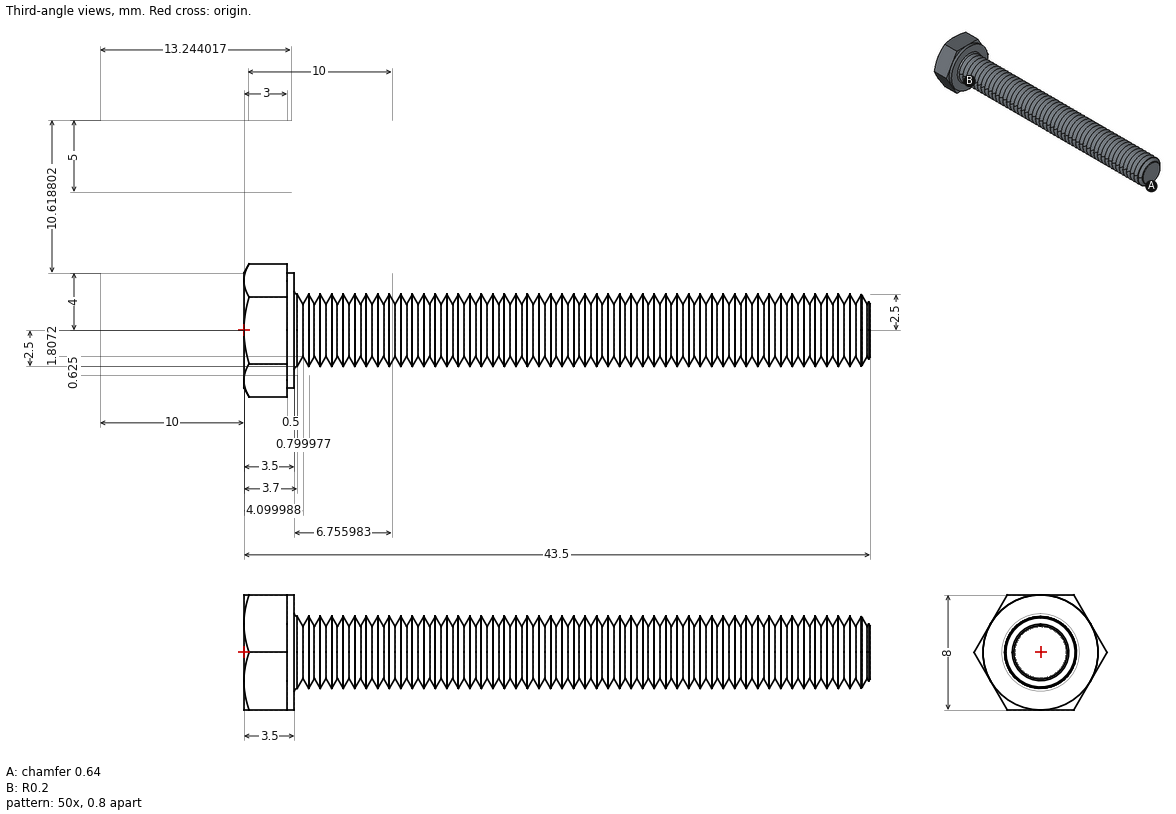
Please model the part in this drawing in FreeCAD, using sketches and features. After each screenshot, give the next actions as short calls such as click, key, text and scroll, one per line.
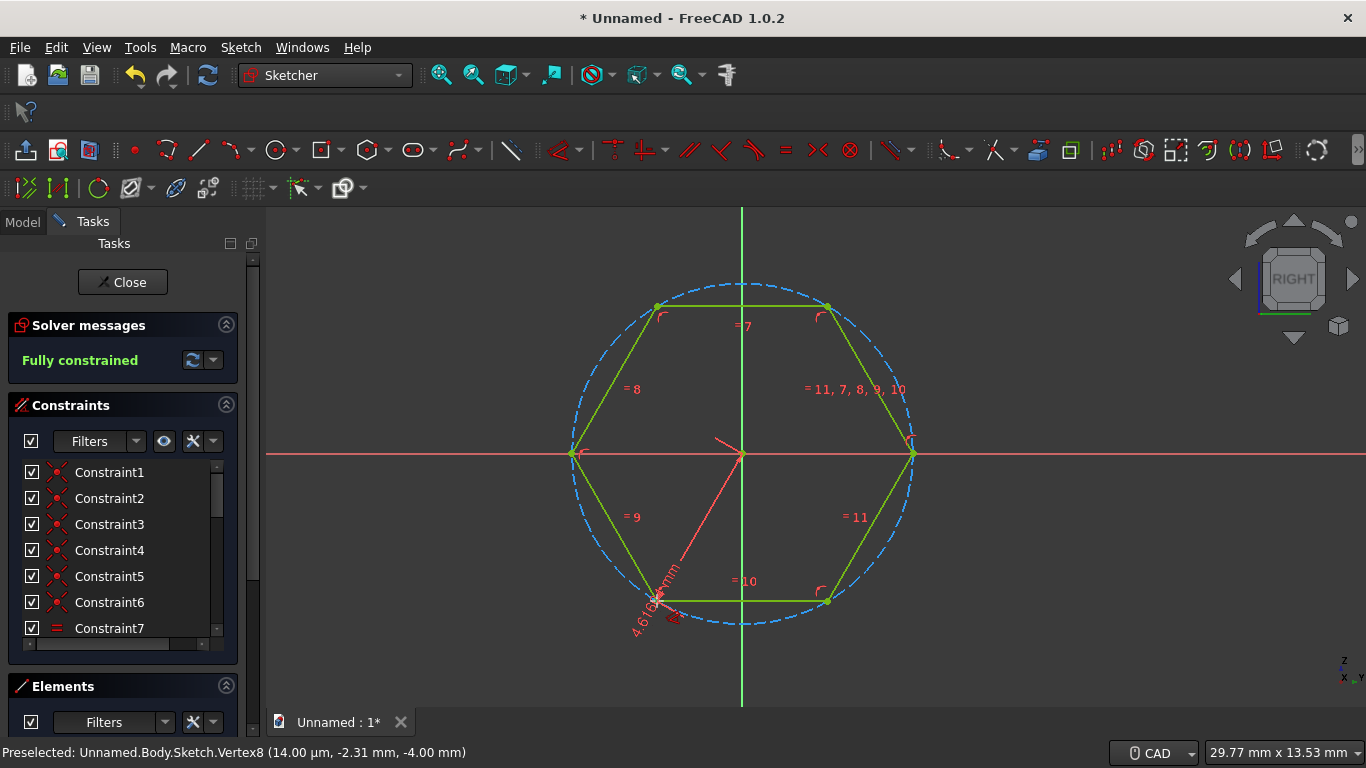
click(828, 306)
click(910, 350)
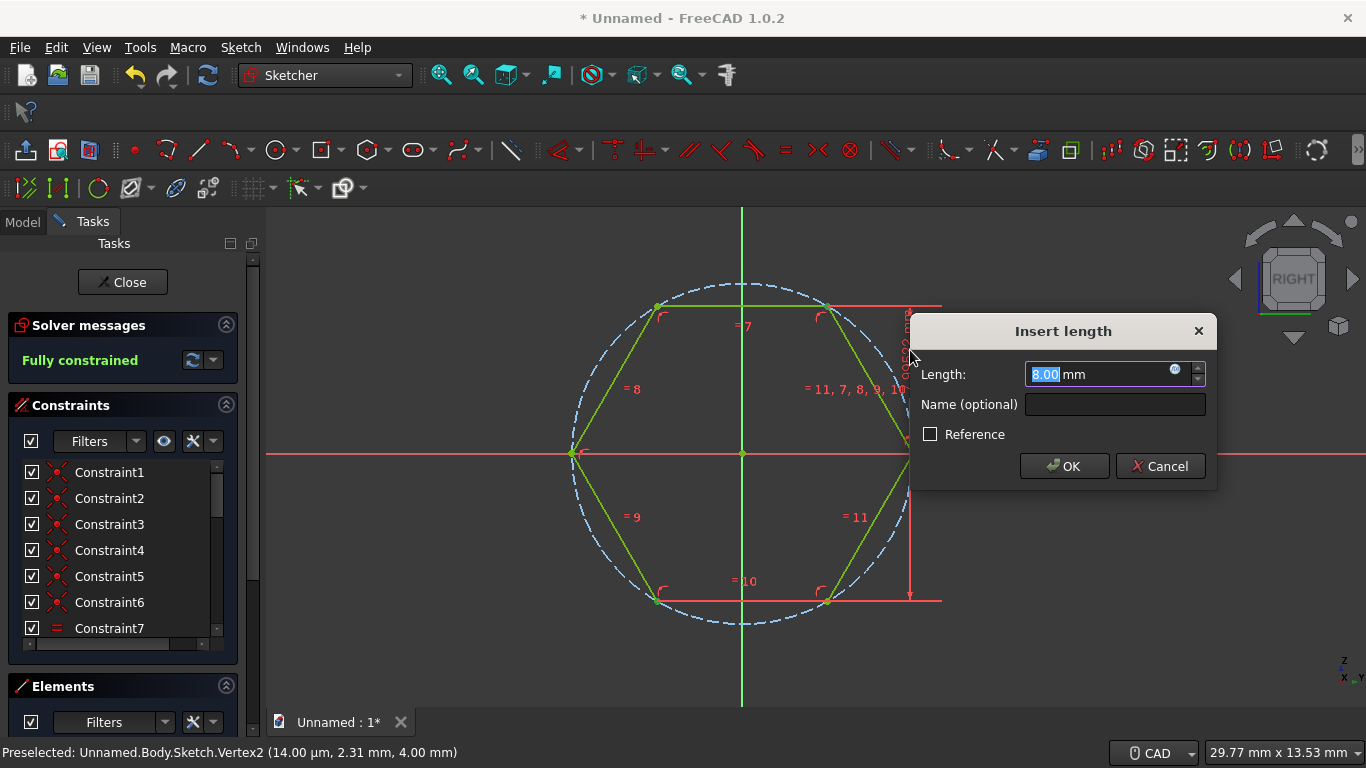
text(8)
key(Return)
key(Escape)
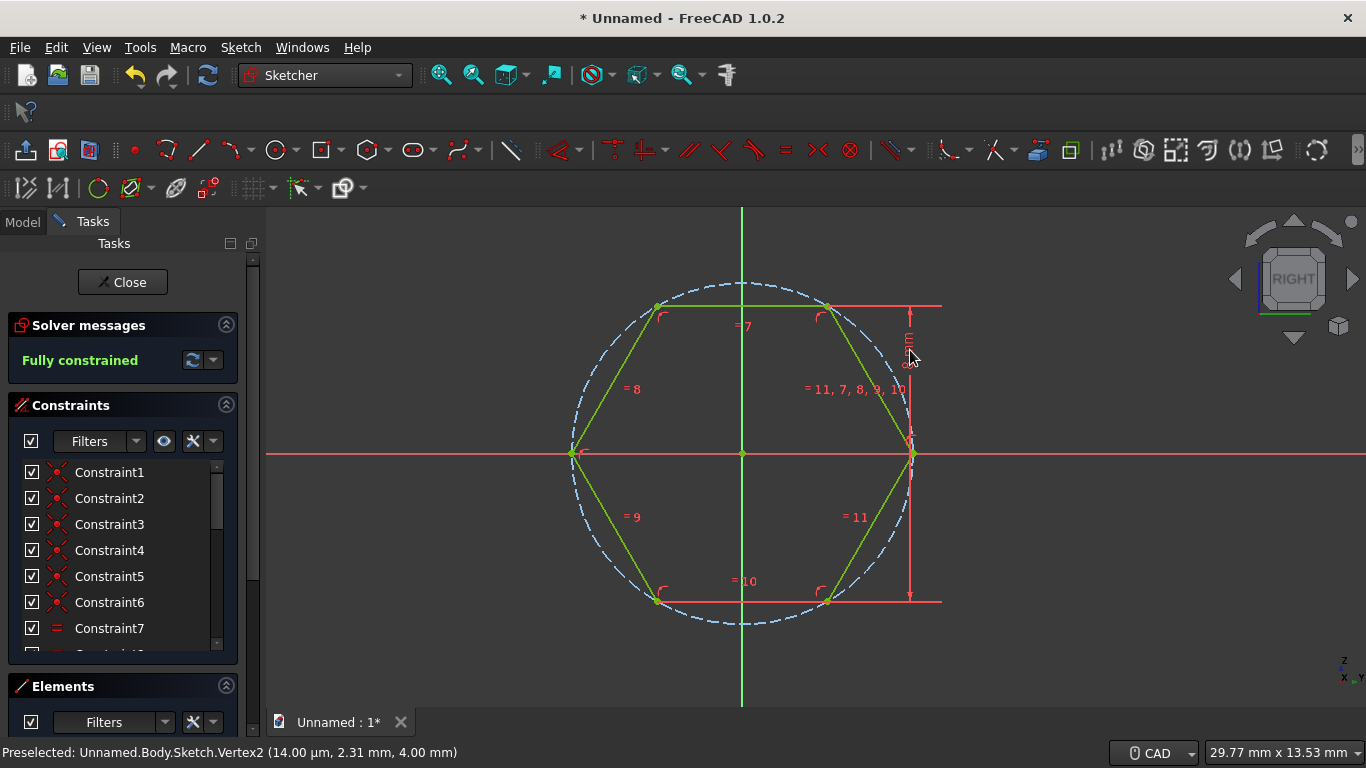
click(123, 282)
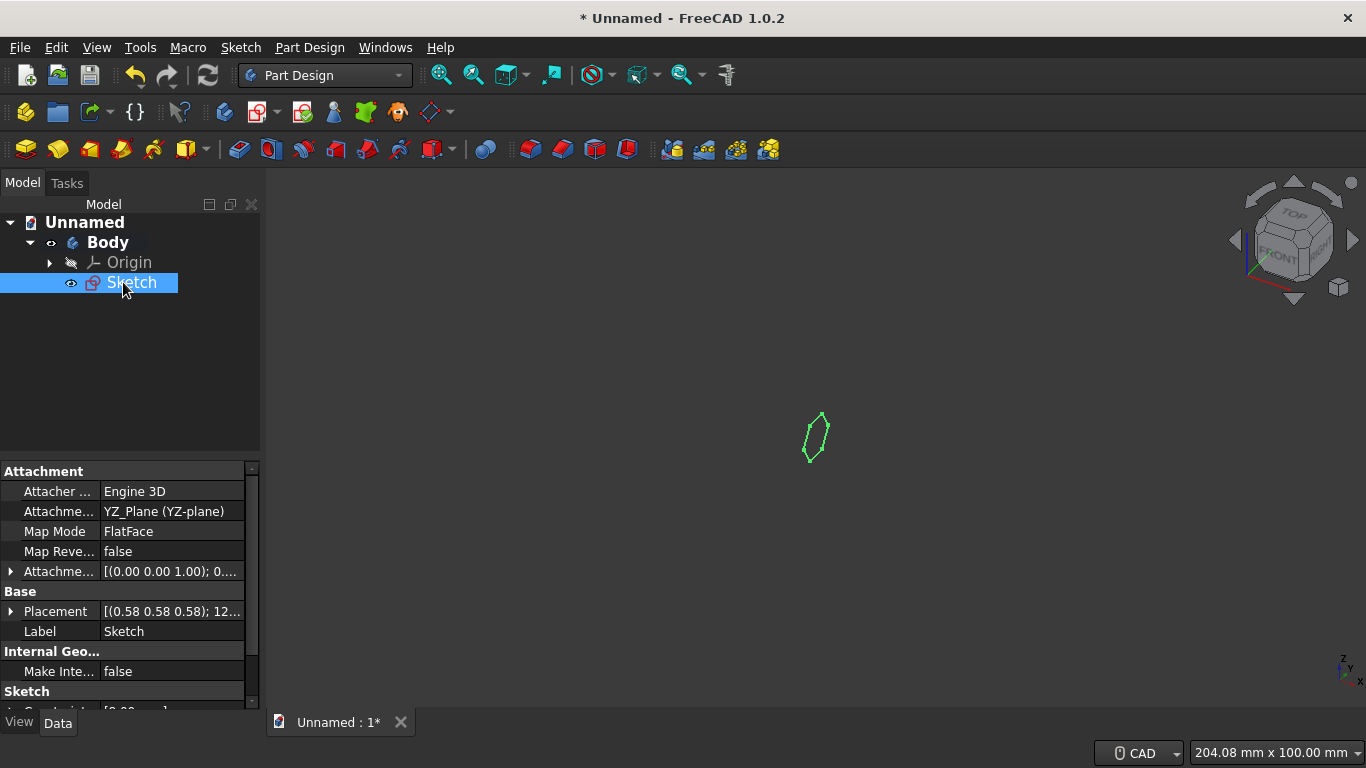
click(26, 150)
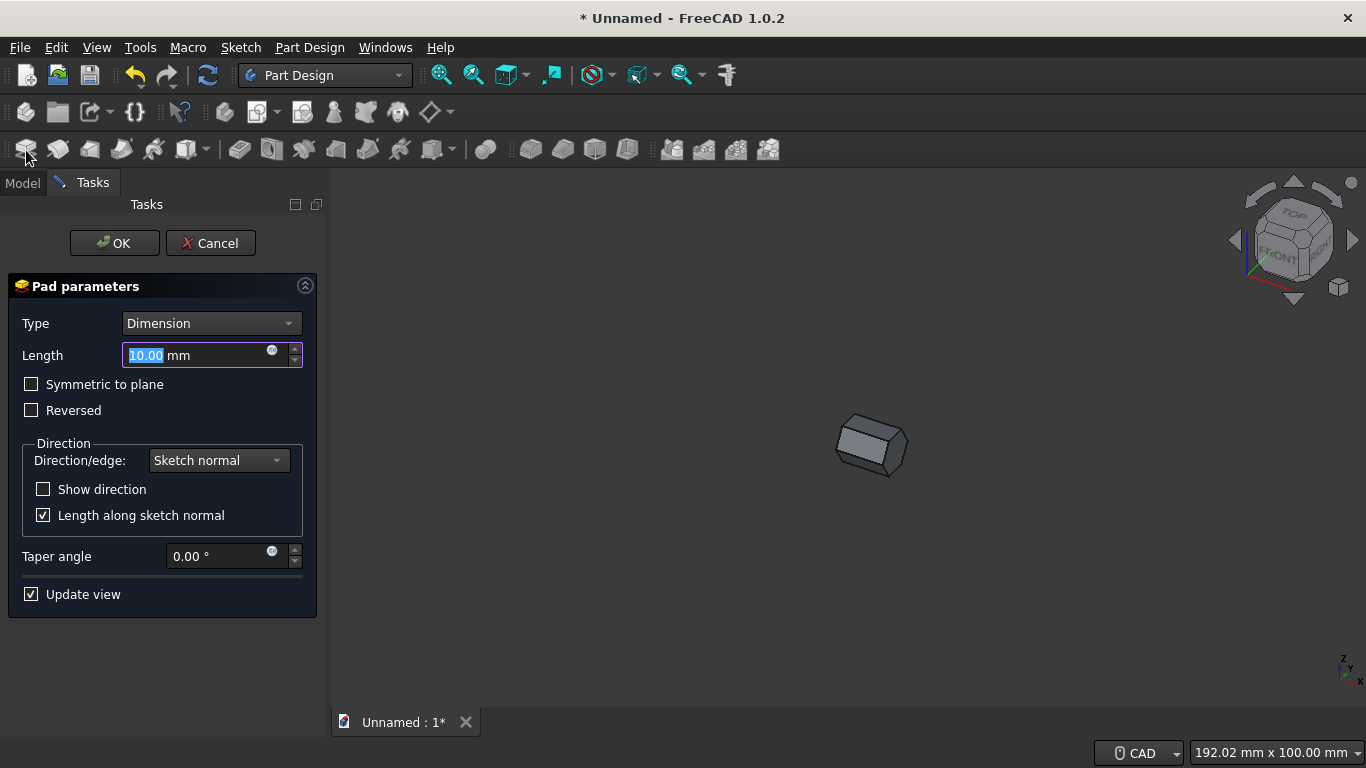
text(3.5)
key(Tab)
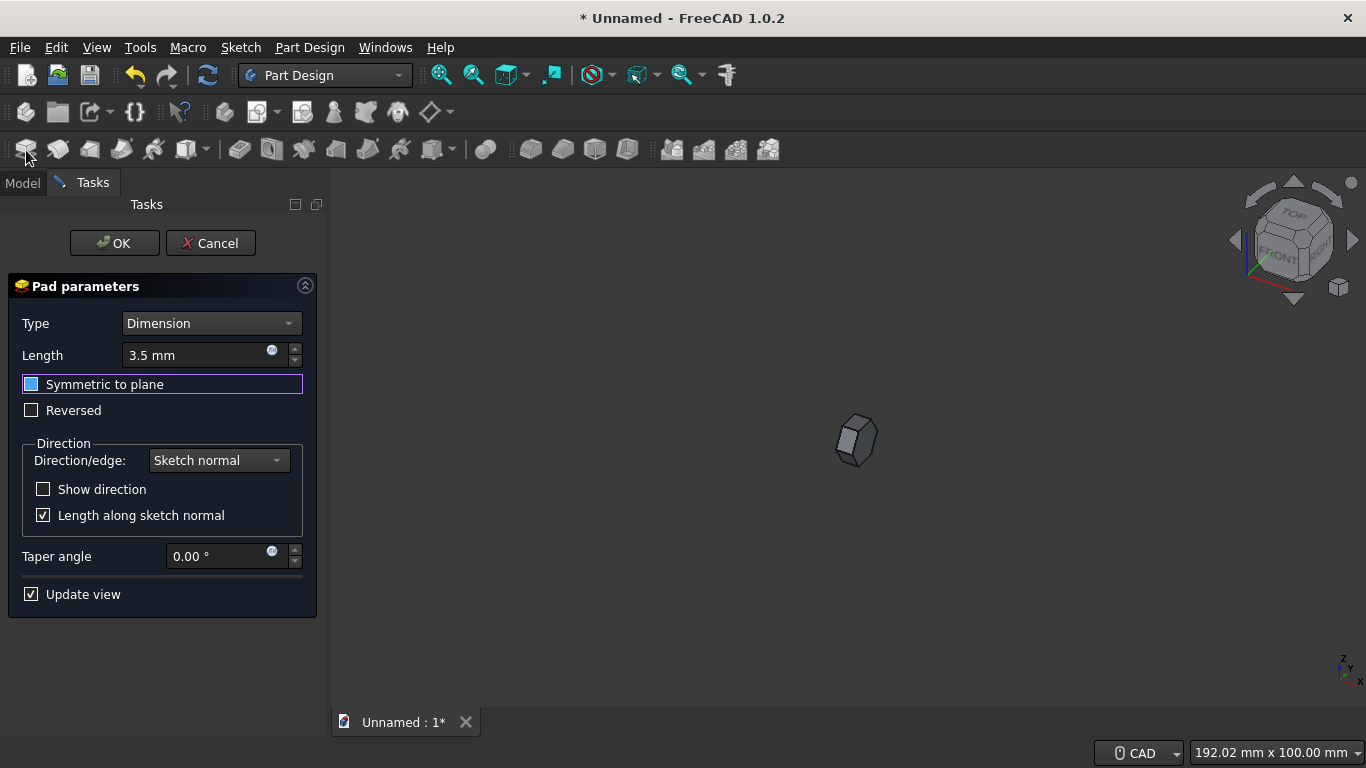
click(115, 243)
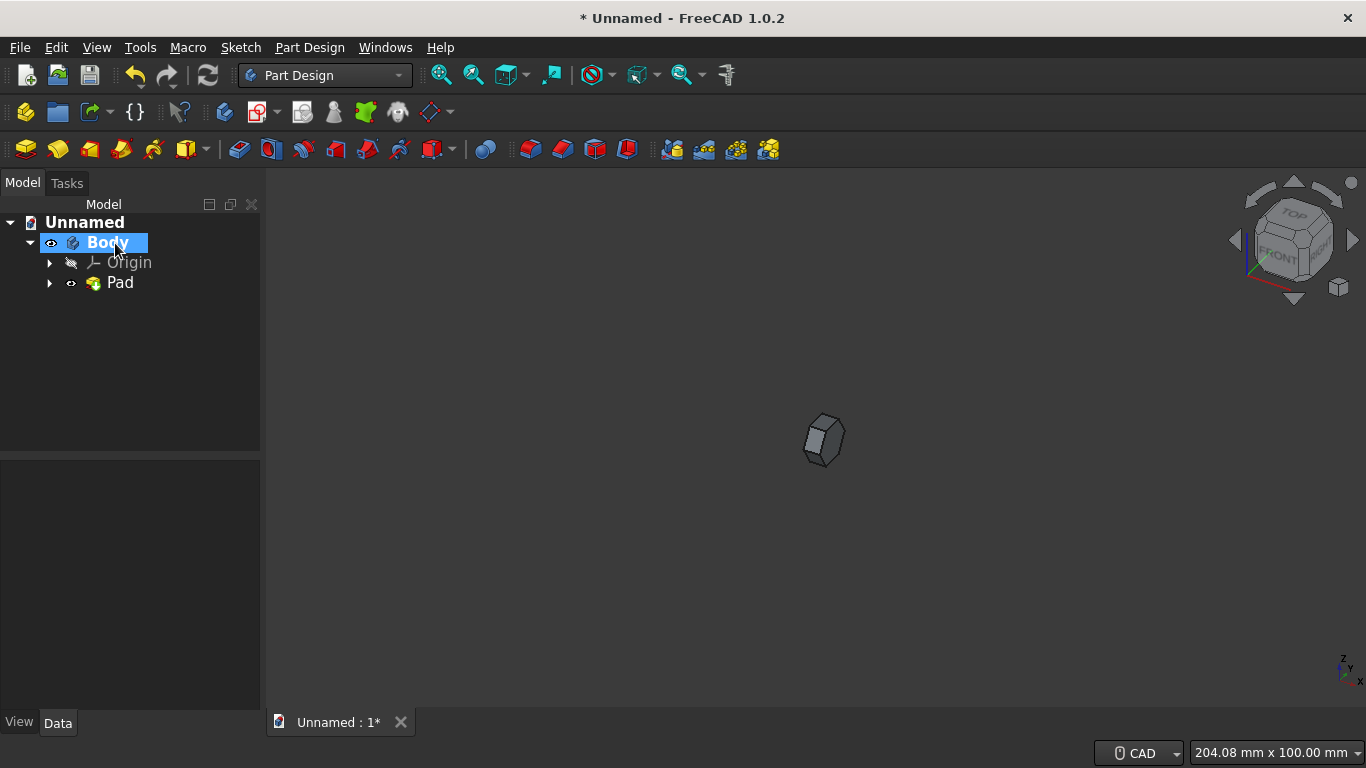
click(442, 76)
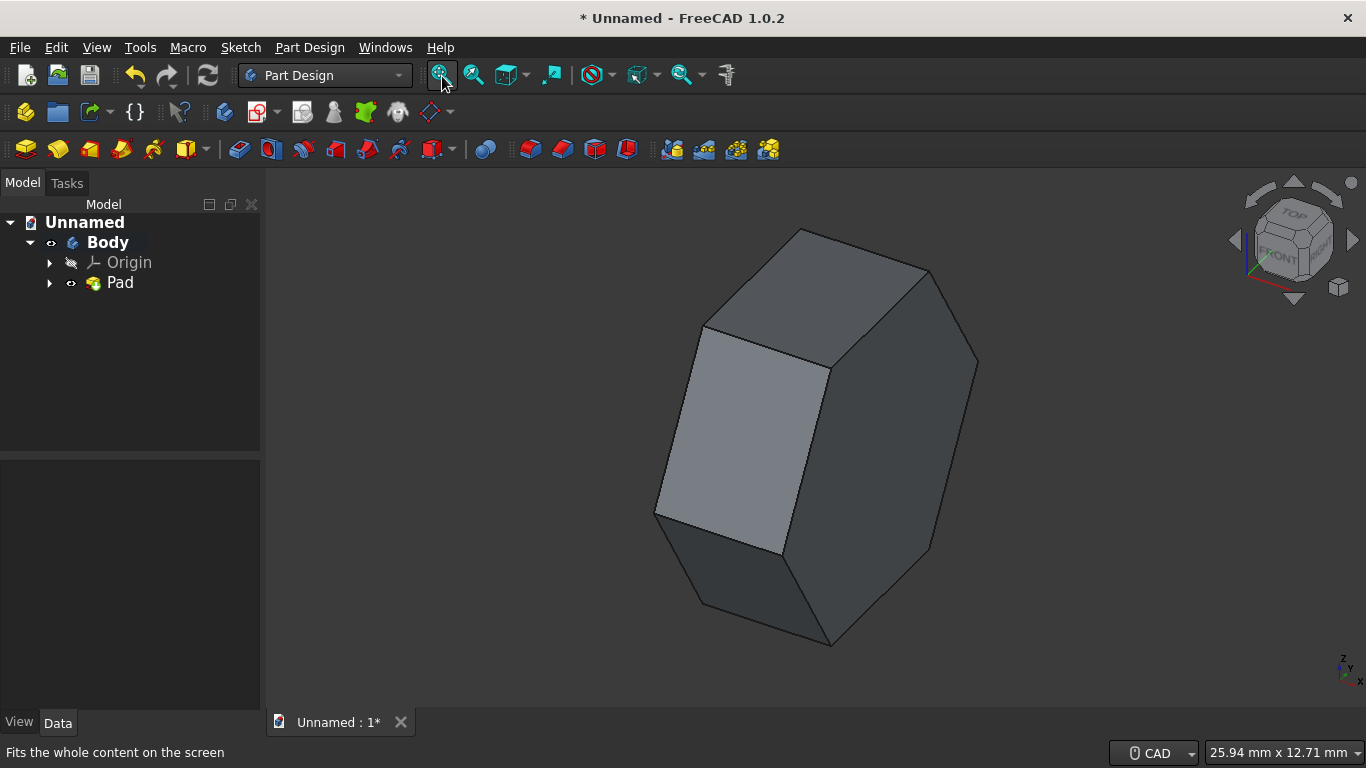
click(258, 112)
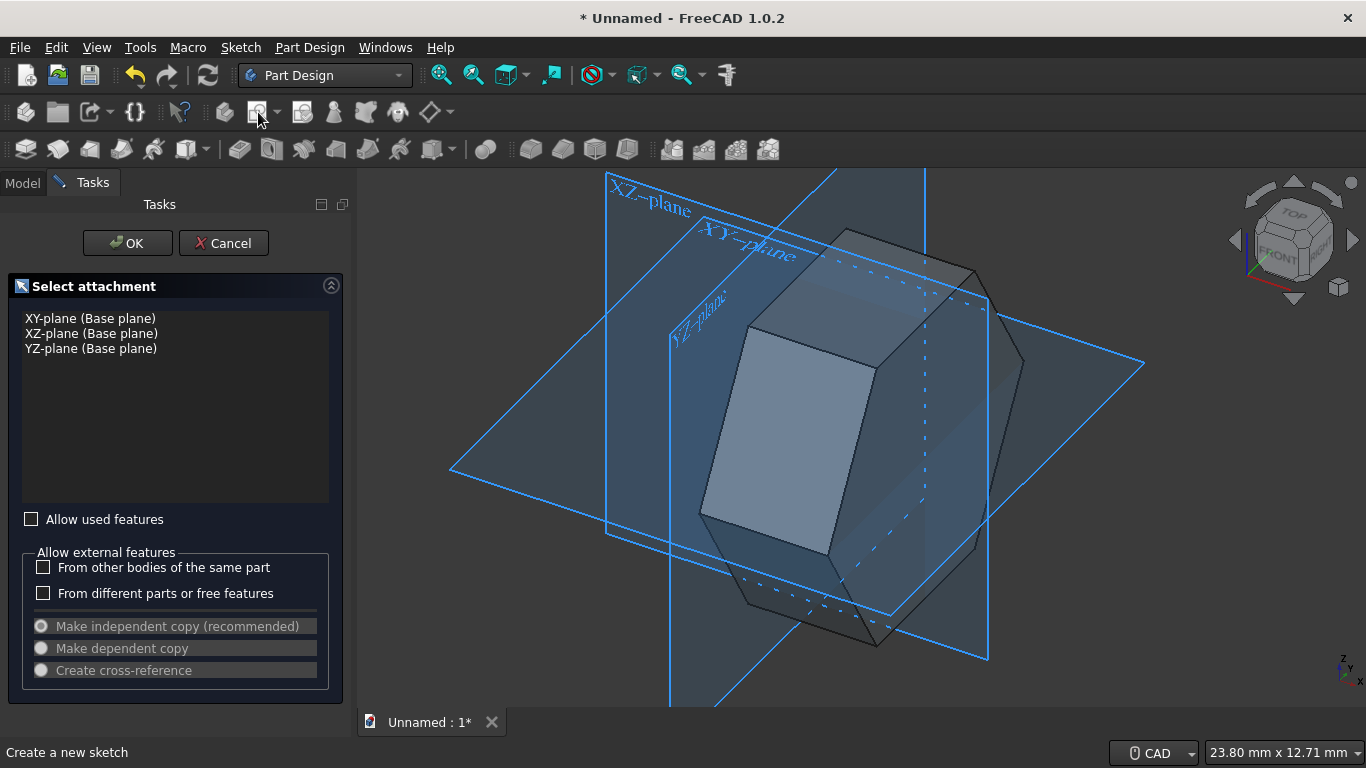
click(82, 318)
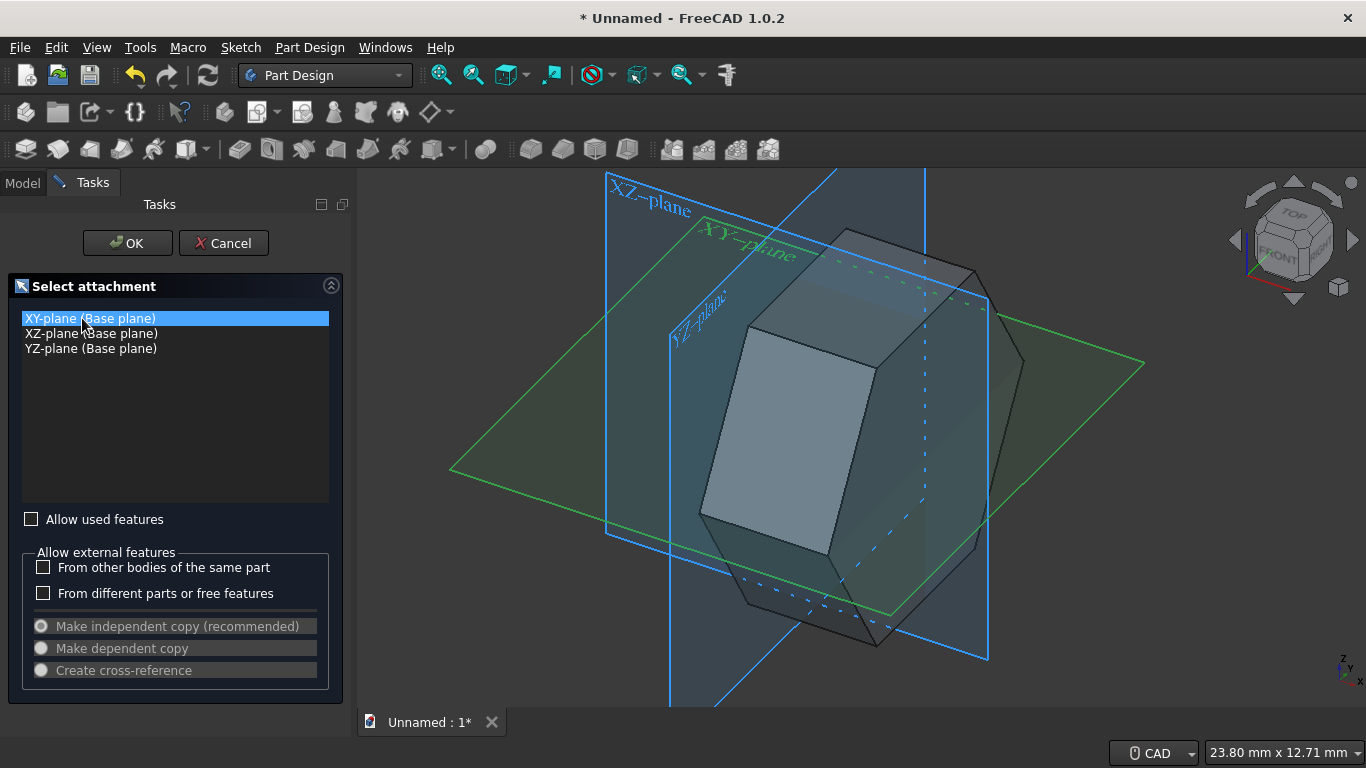
click(128, 243)